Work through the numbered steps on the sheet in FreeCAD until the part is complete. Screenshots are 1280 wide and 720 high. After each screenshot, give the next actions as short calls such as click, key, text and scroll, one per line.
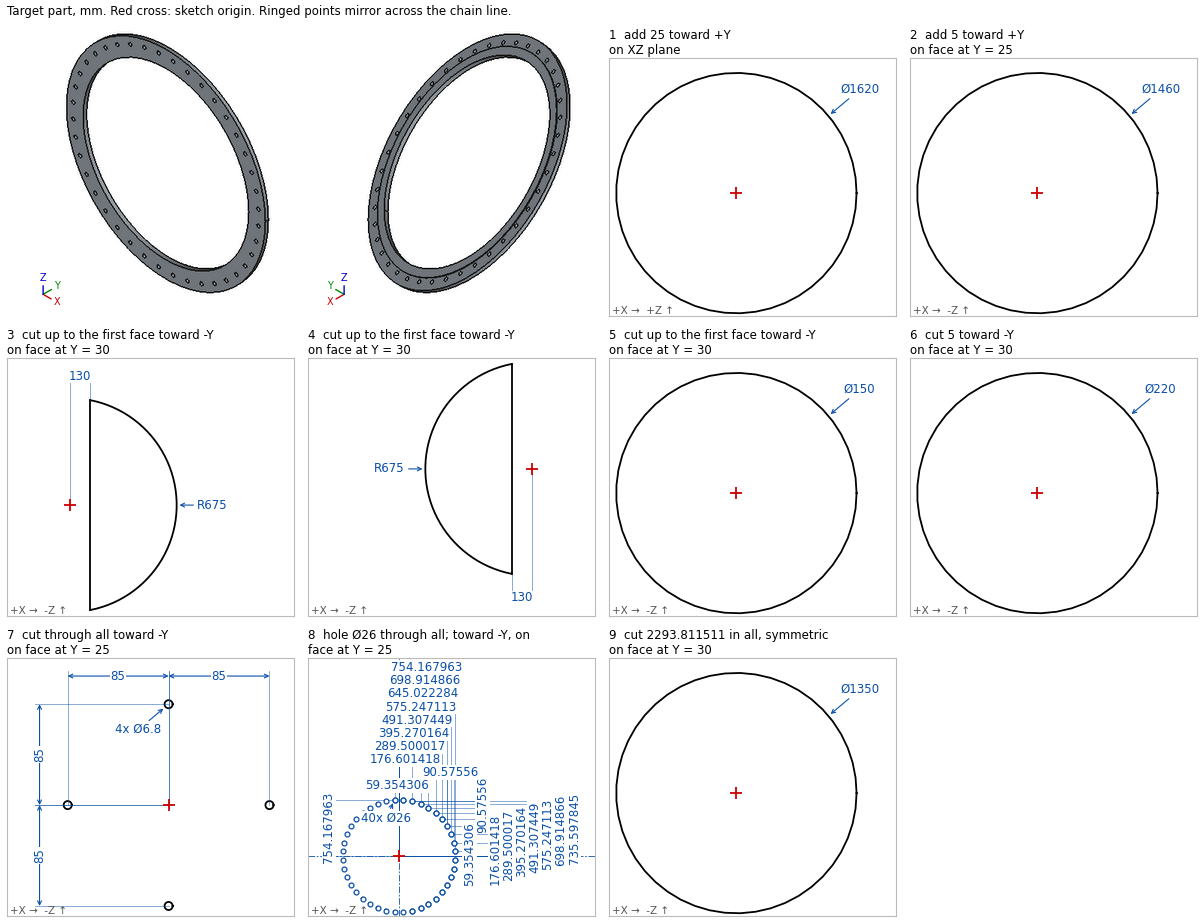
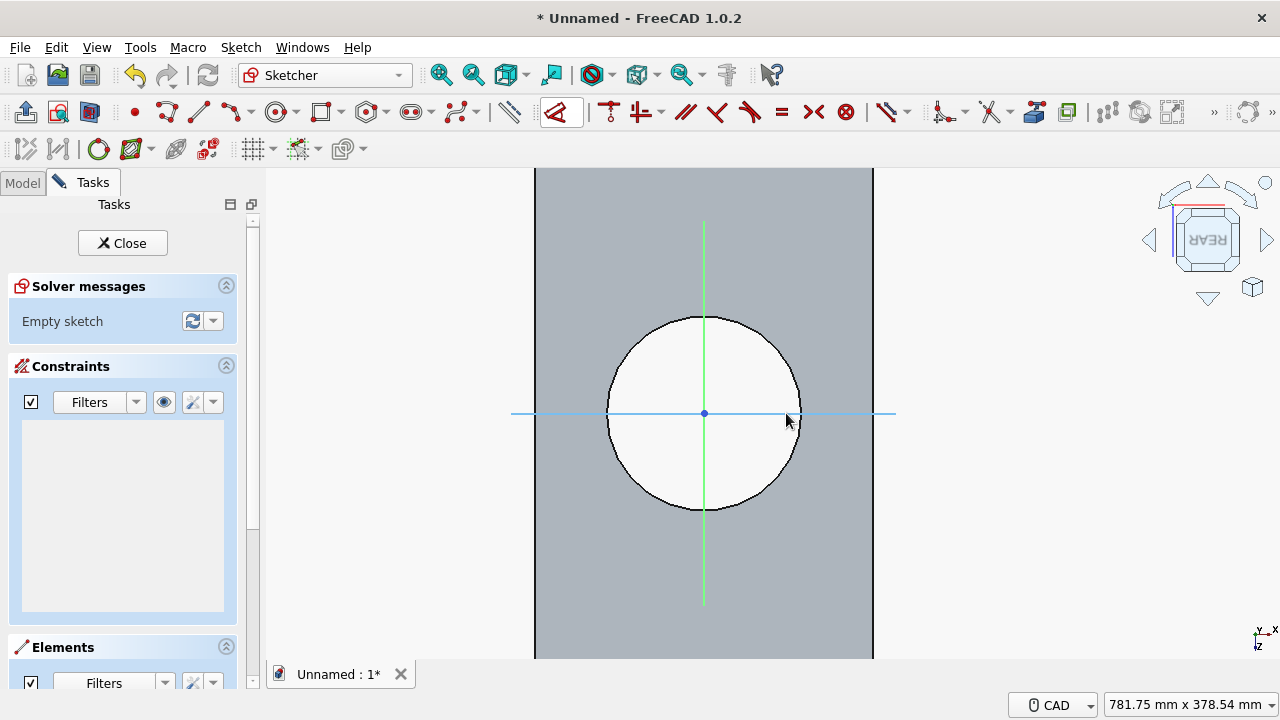
click(276, 112)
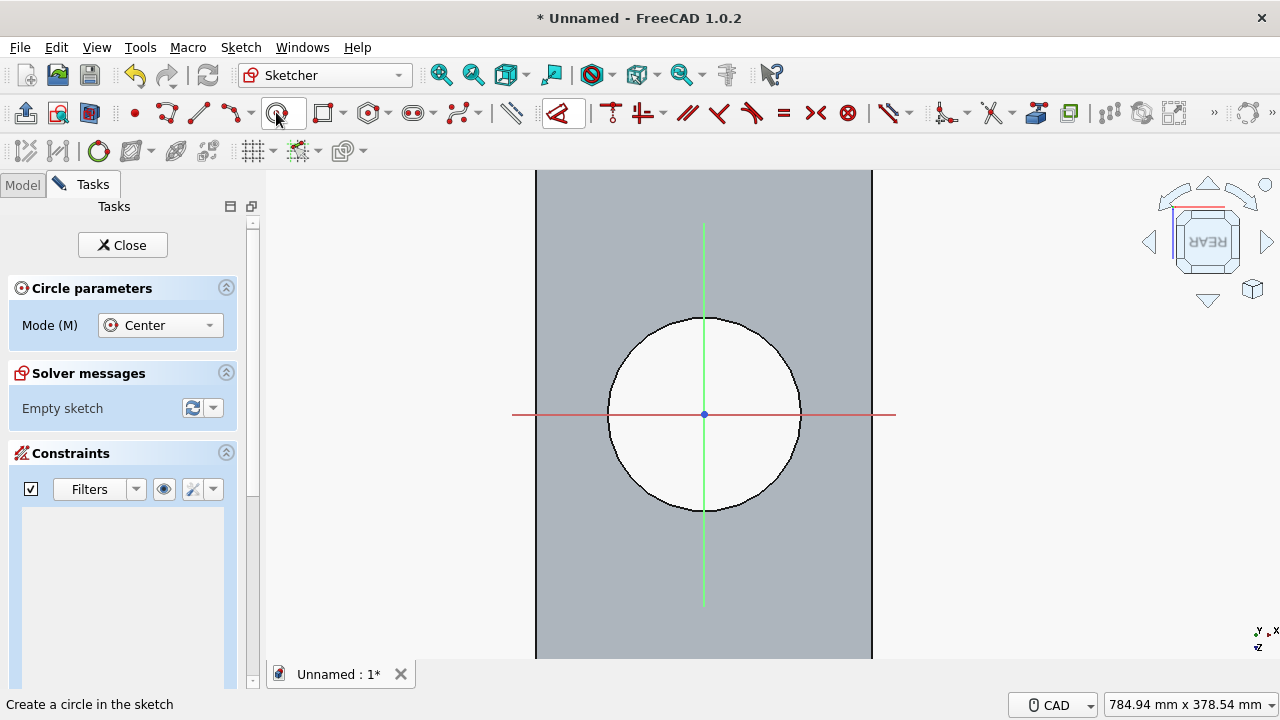
click(704, 414)
click(805, 314)
key(Escape)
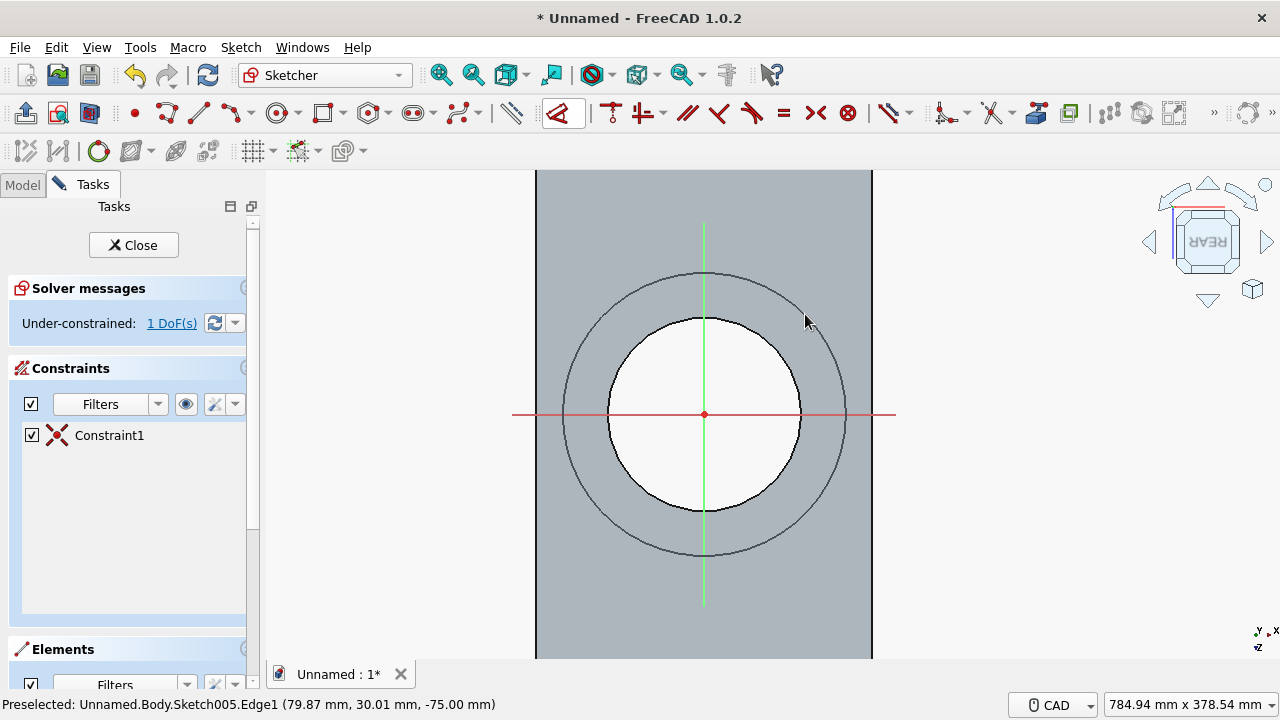
click(804, 314)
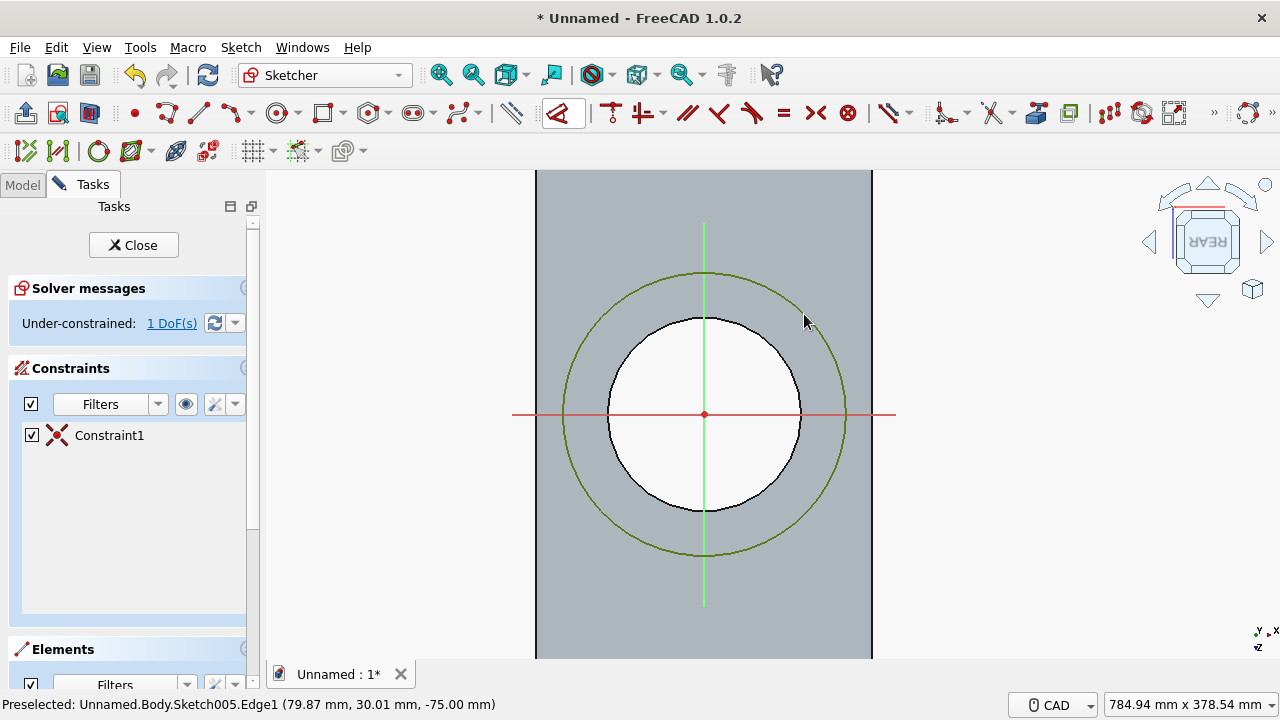
click(580, 114)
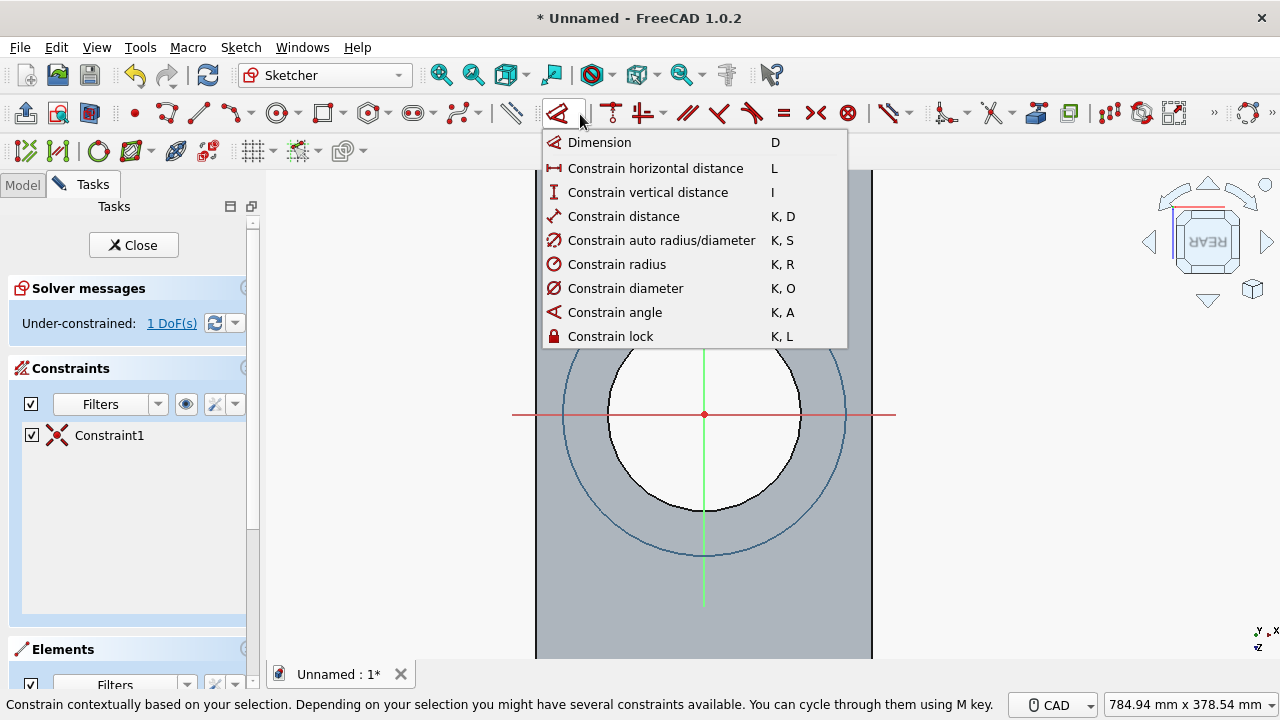
click(695, 288)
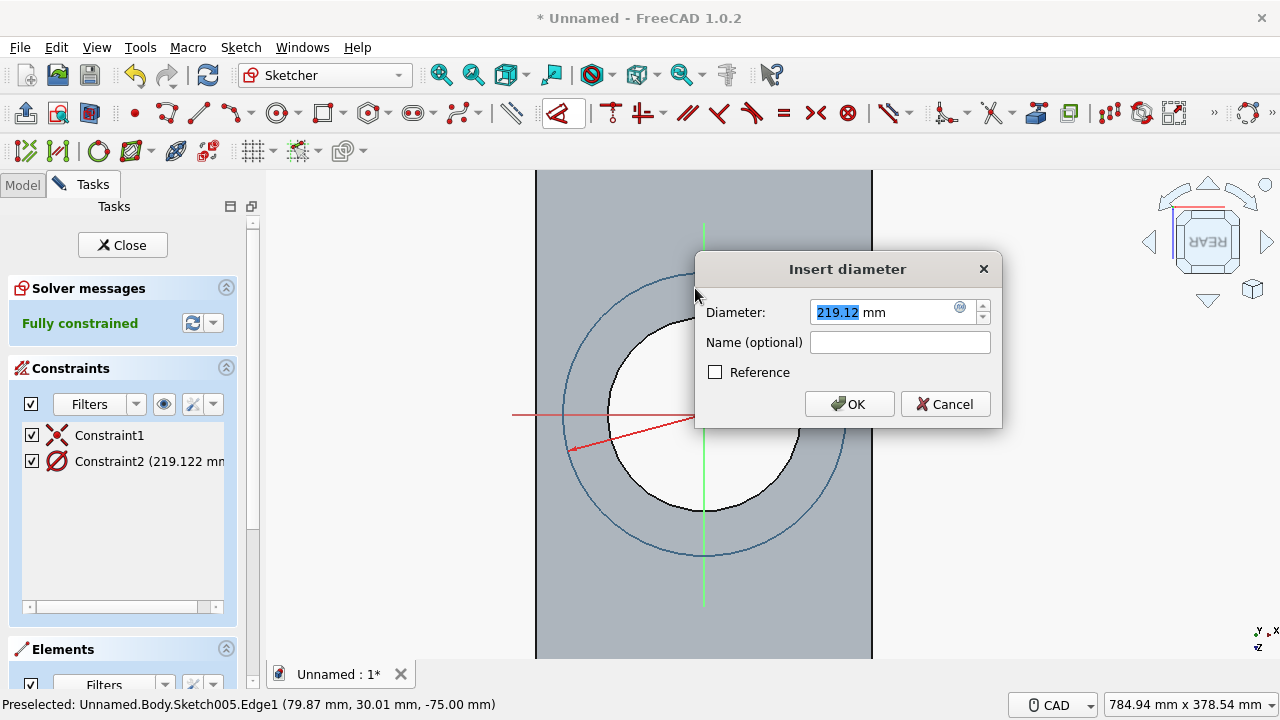
text(220)
key(Return)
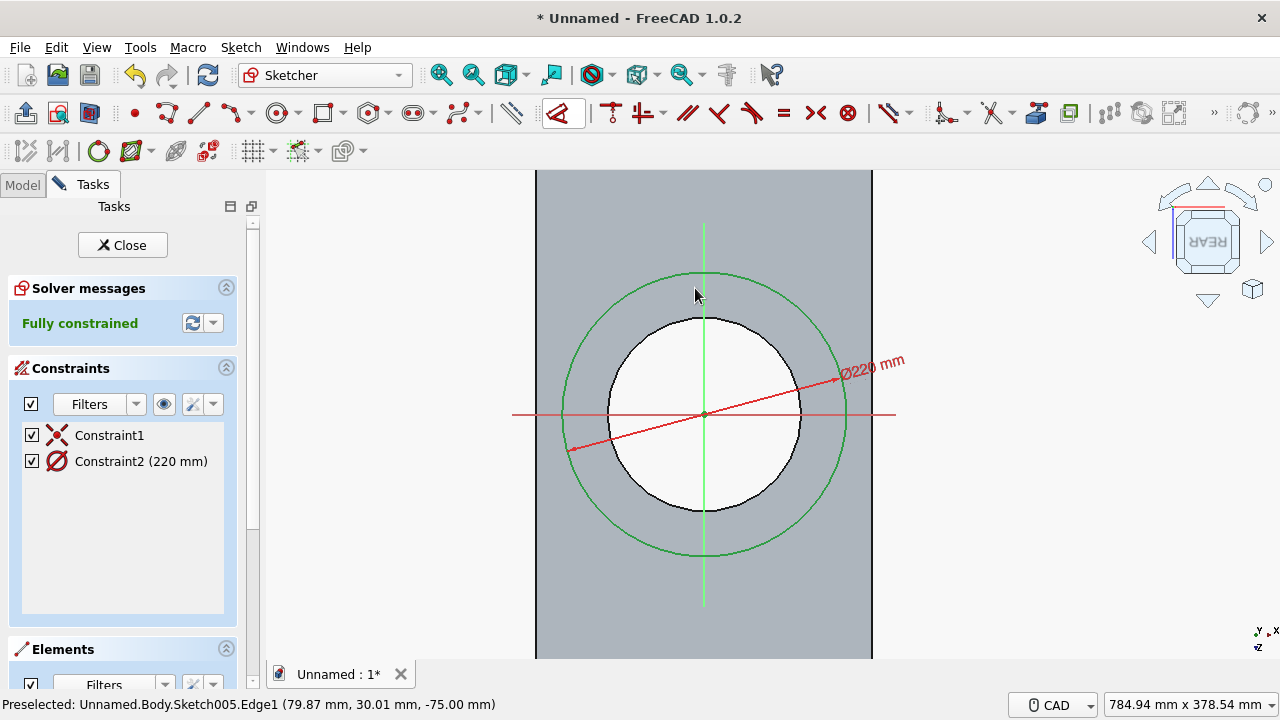
click(123, 245)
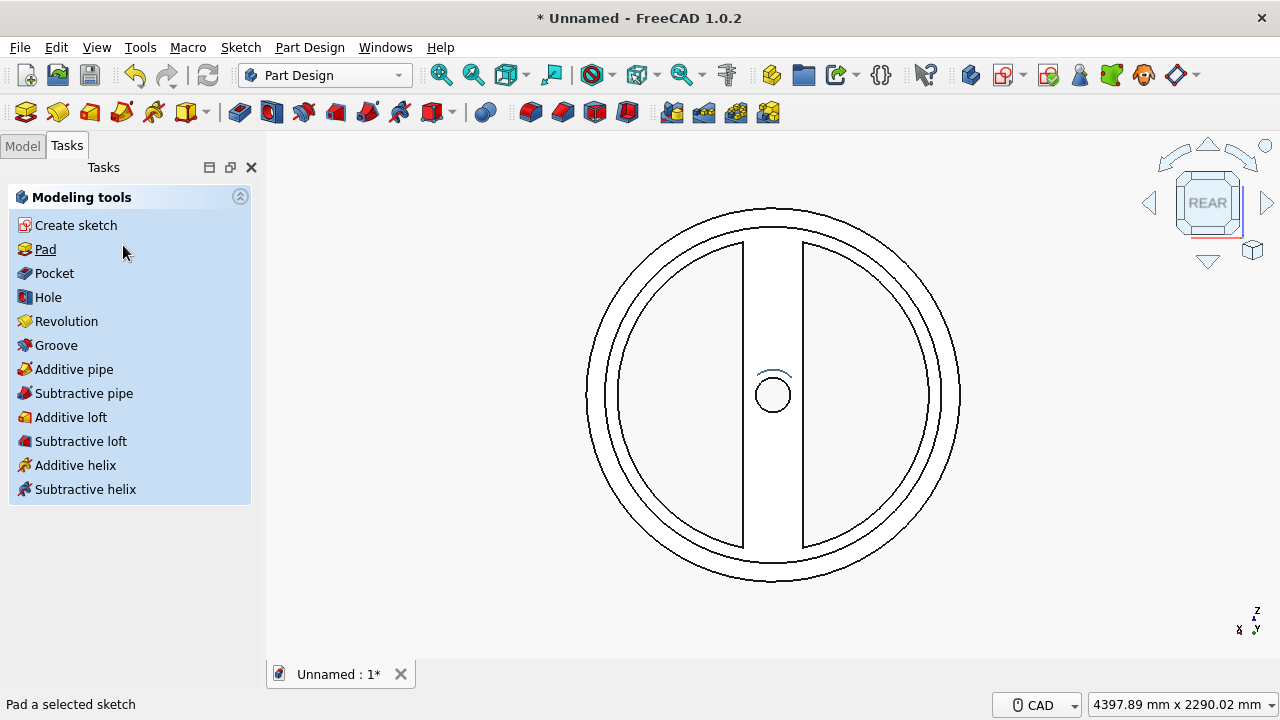
click(240, 112)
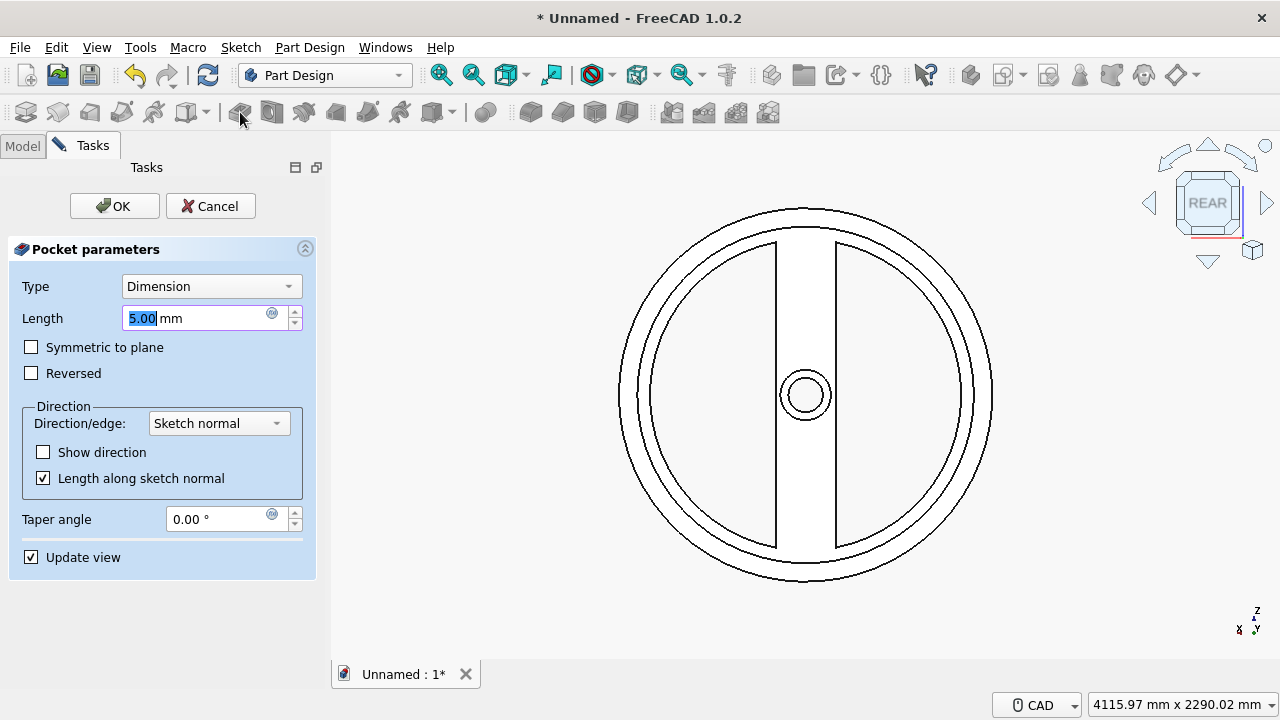
text(5)
key(Tab)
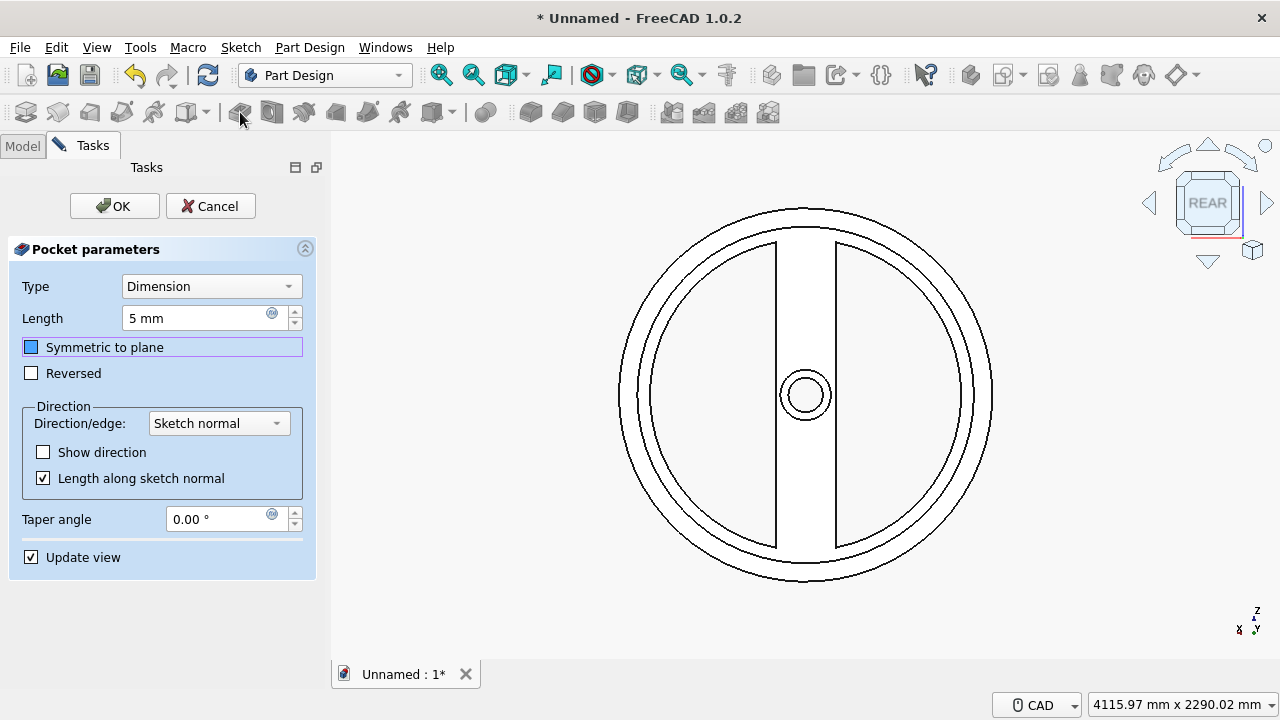
click(115, 206)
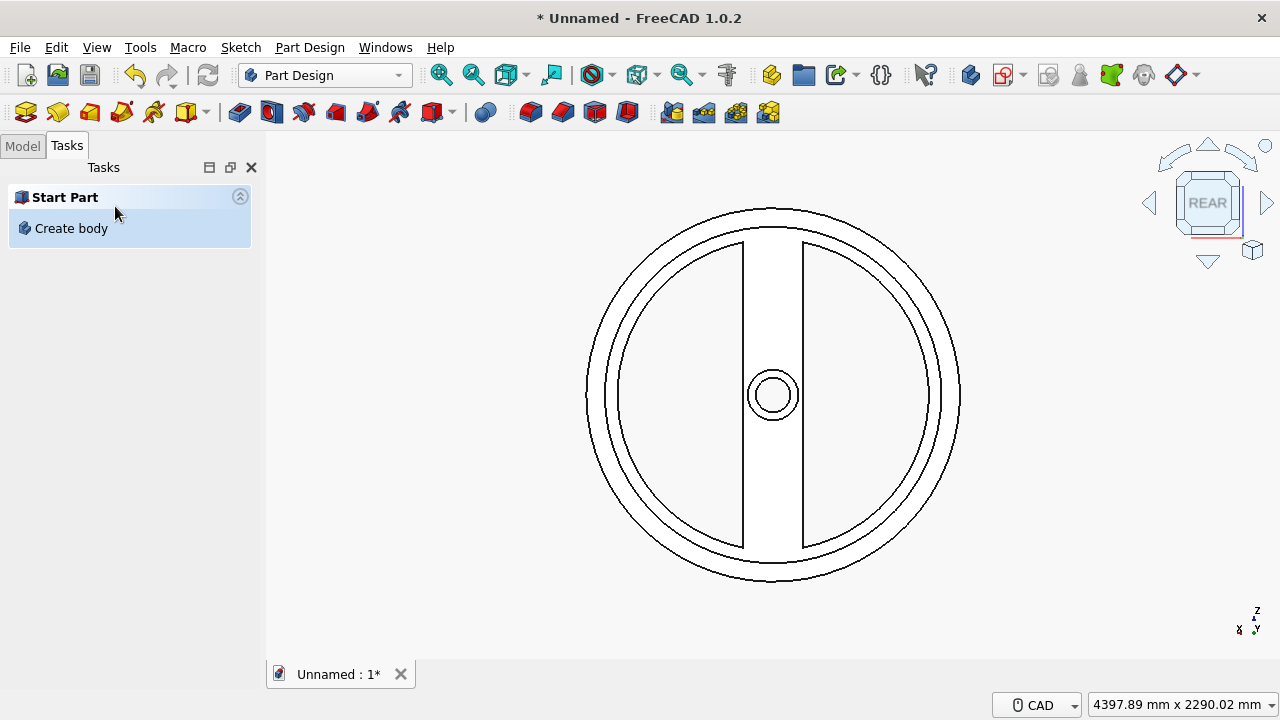
scroll(826, 554, up, 15)